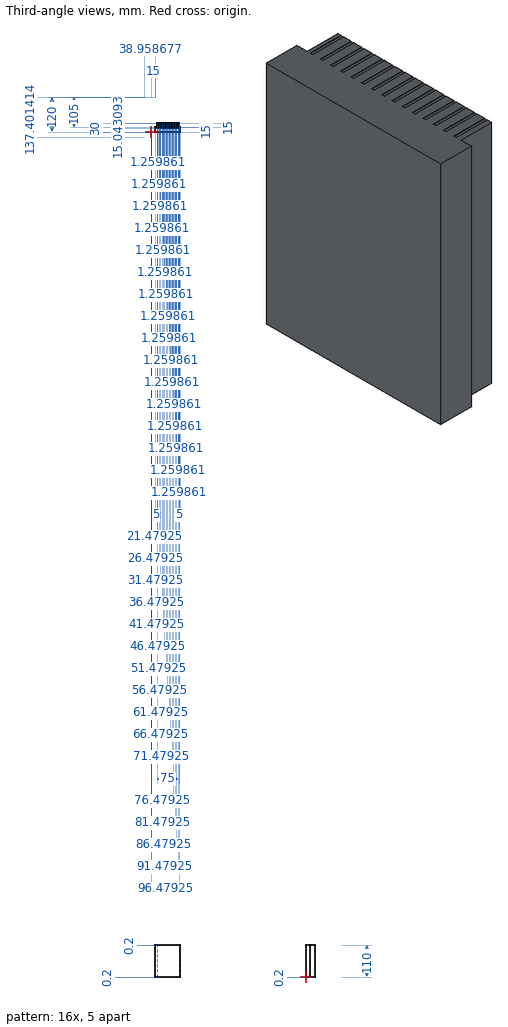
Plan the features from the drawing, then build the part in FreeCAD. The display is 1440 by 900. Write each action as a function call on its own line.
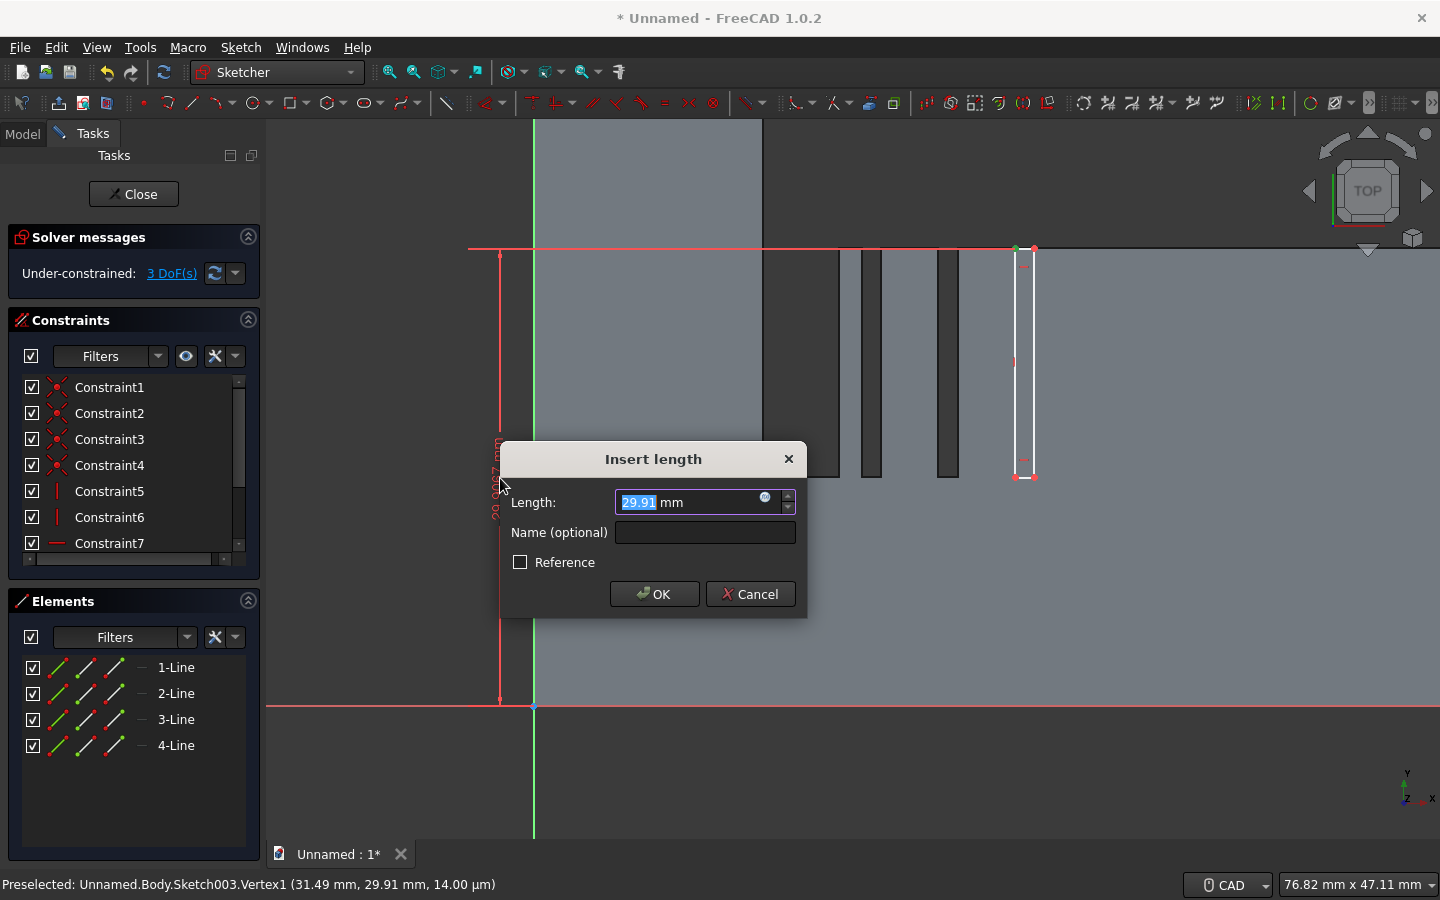
text(30)
key(Return)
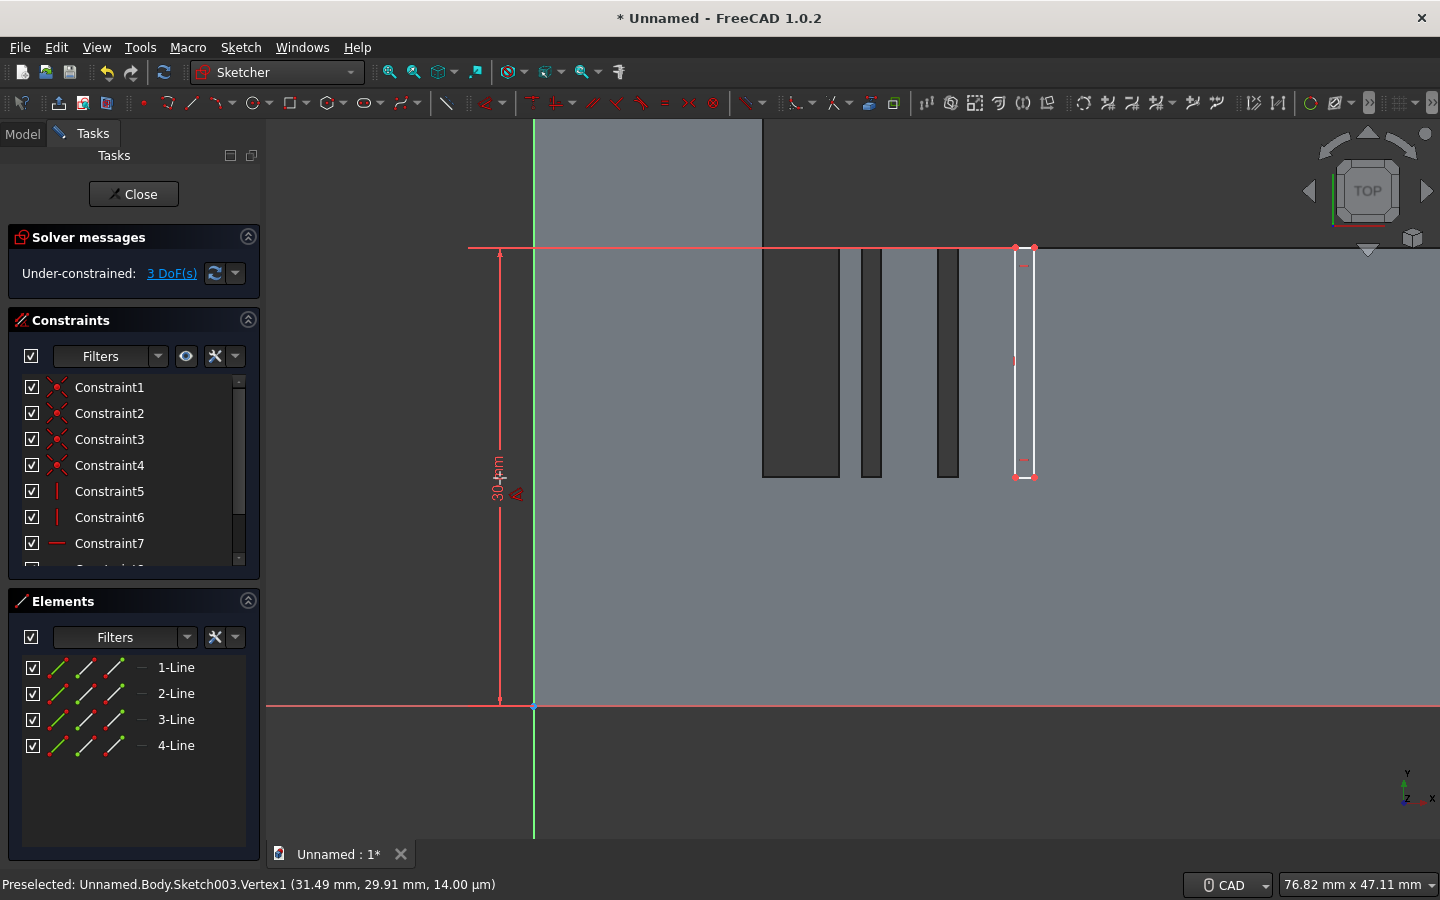
scroll(1025, 478, up, 4)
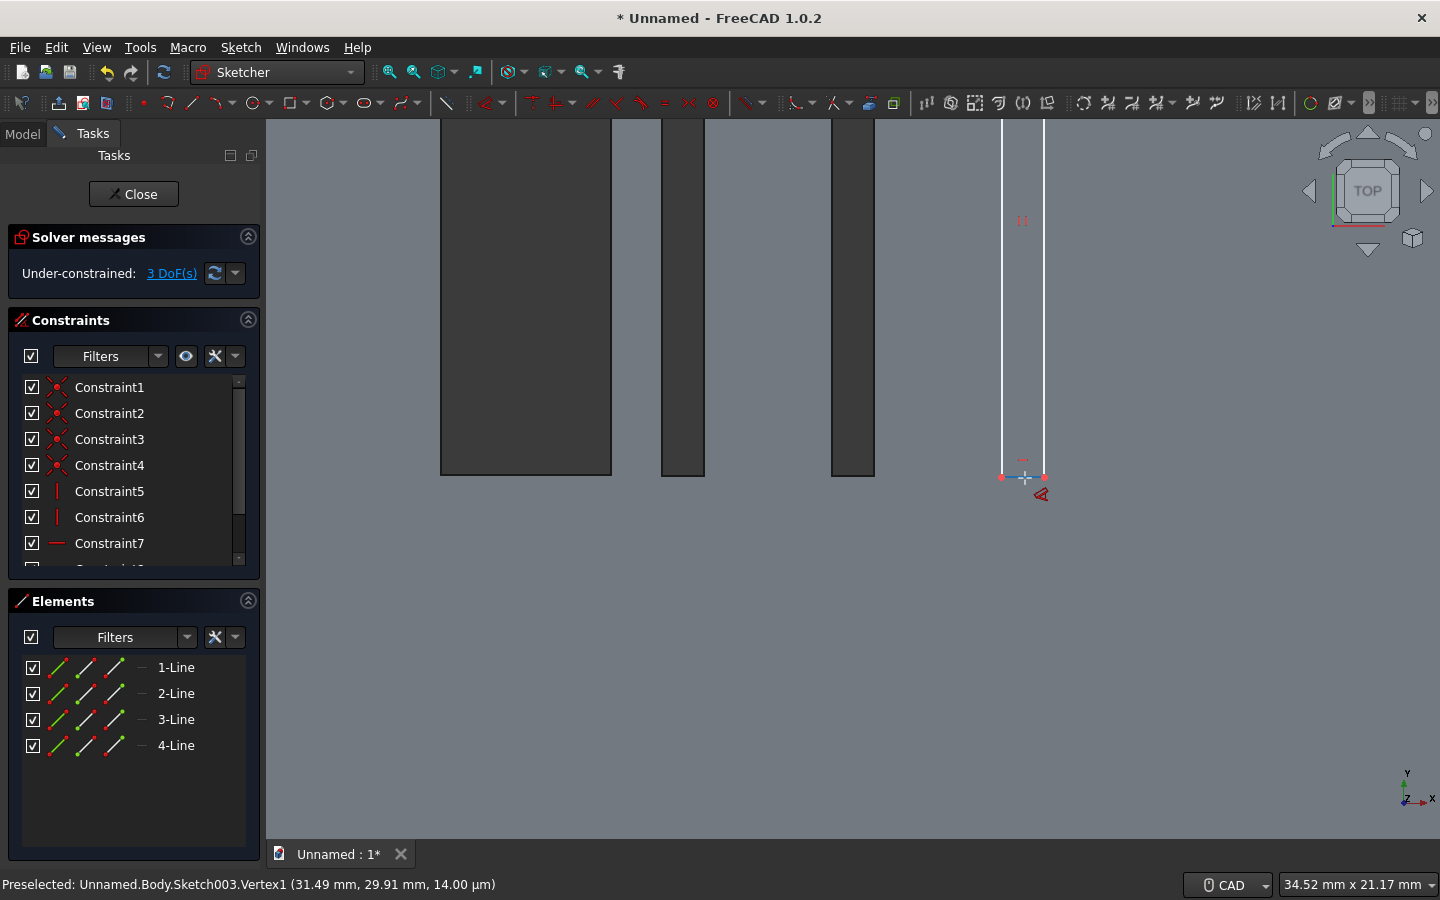
click(1023, 477)
click(1023, 511)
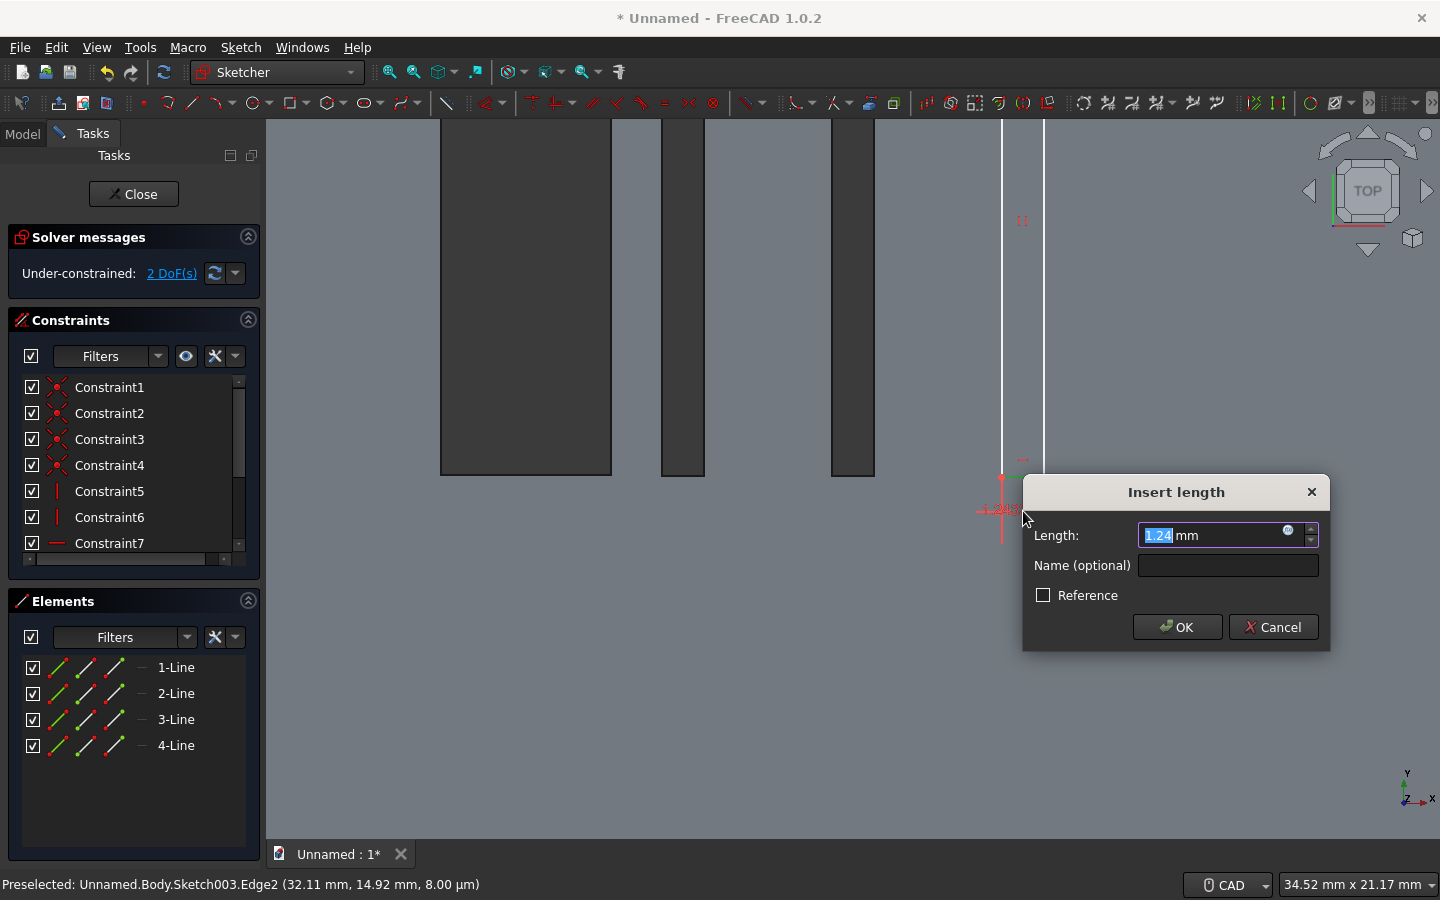
text(1.259861)
key(Return)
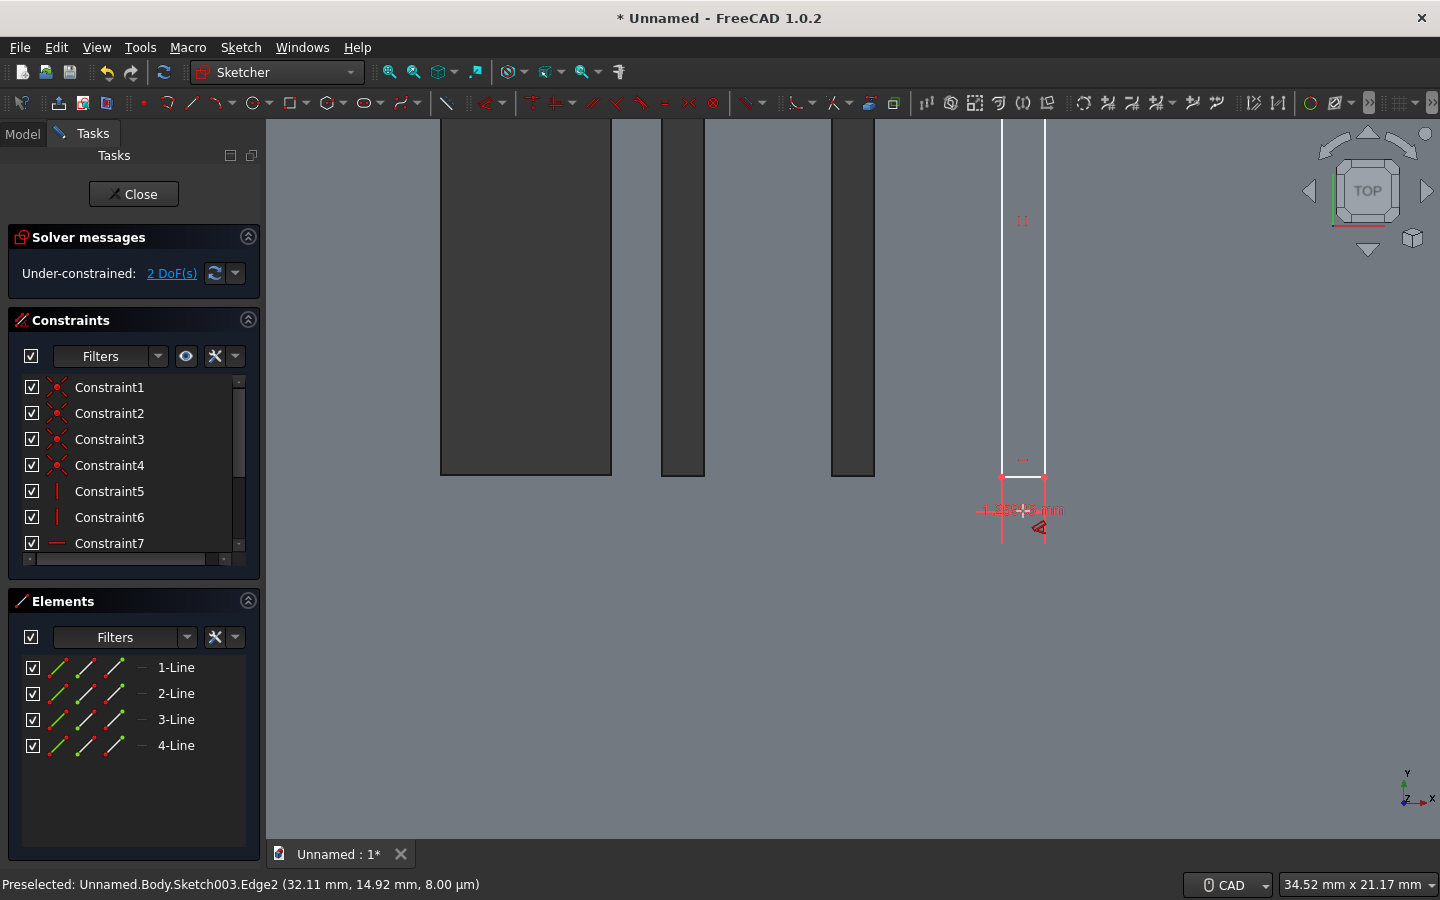
click(1002, 324)
click(968, 312)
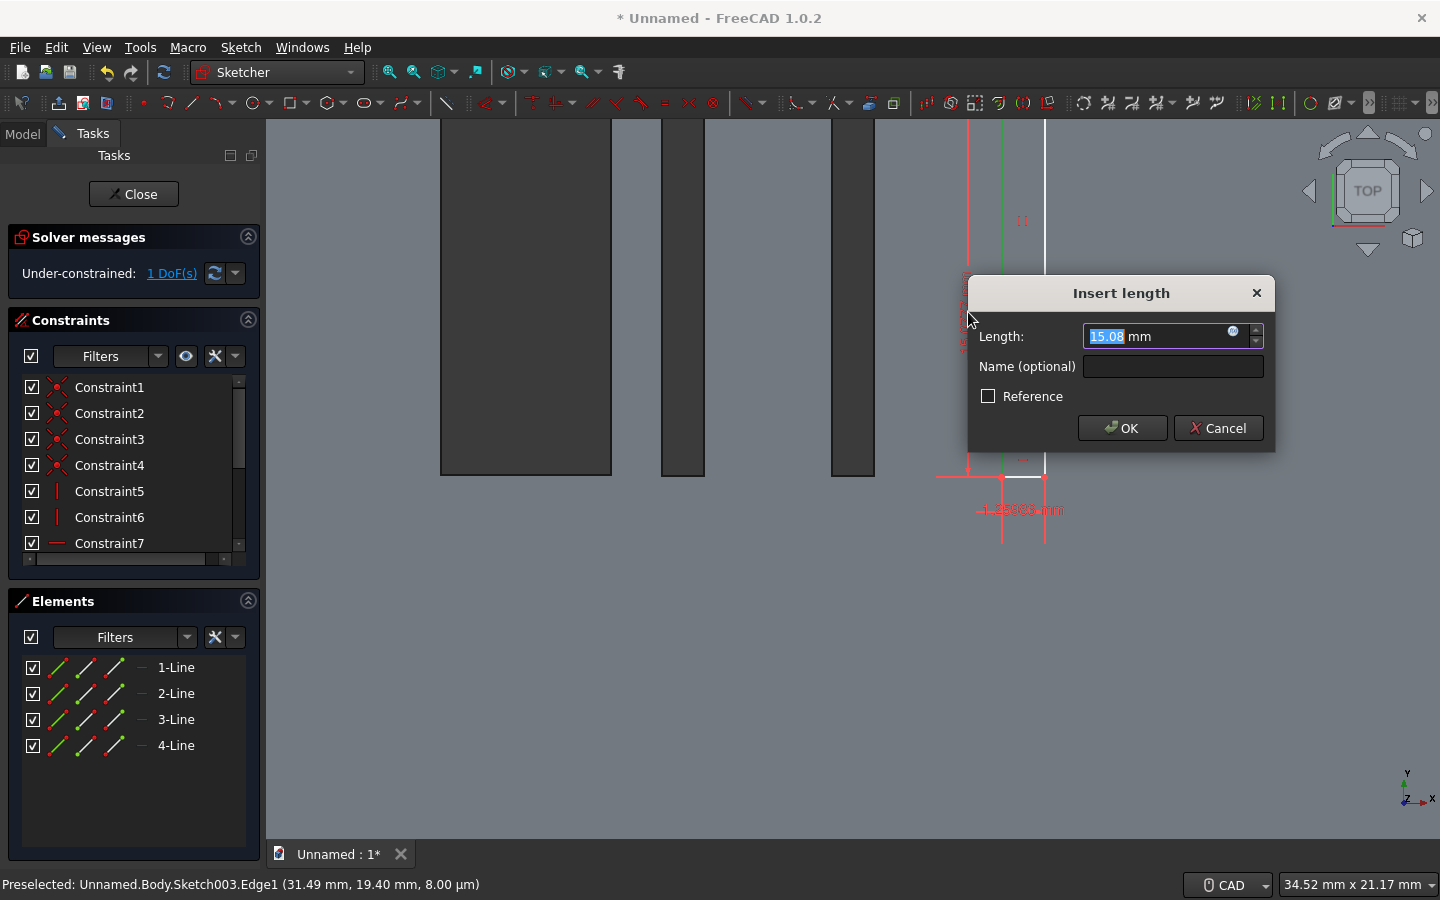
text(15.043093)
key(Return)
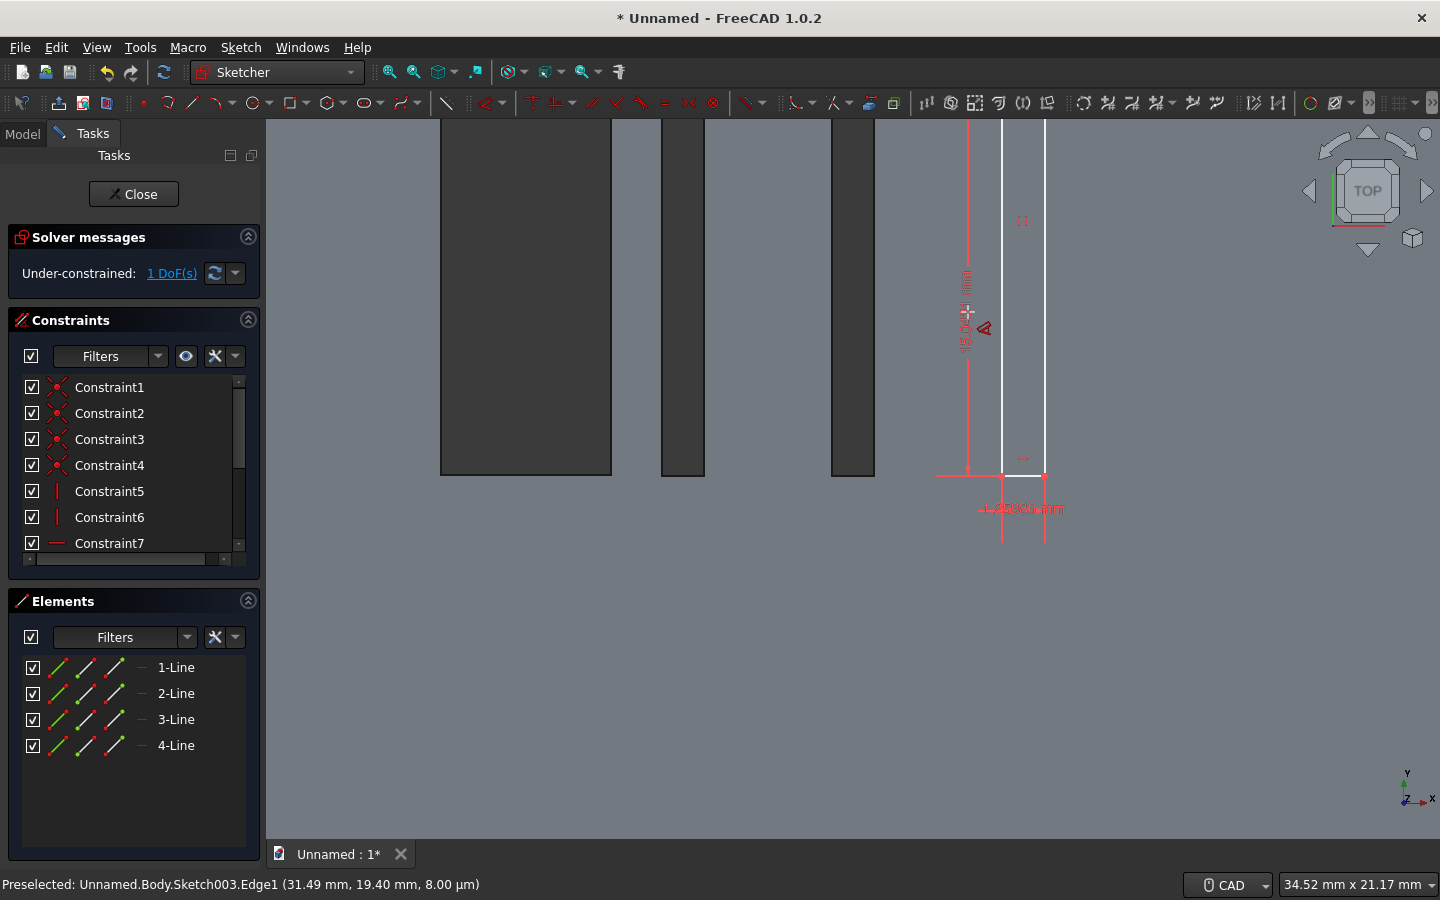
scroll(1027, 482, down, 4)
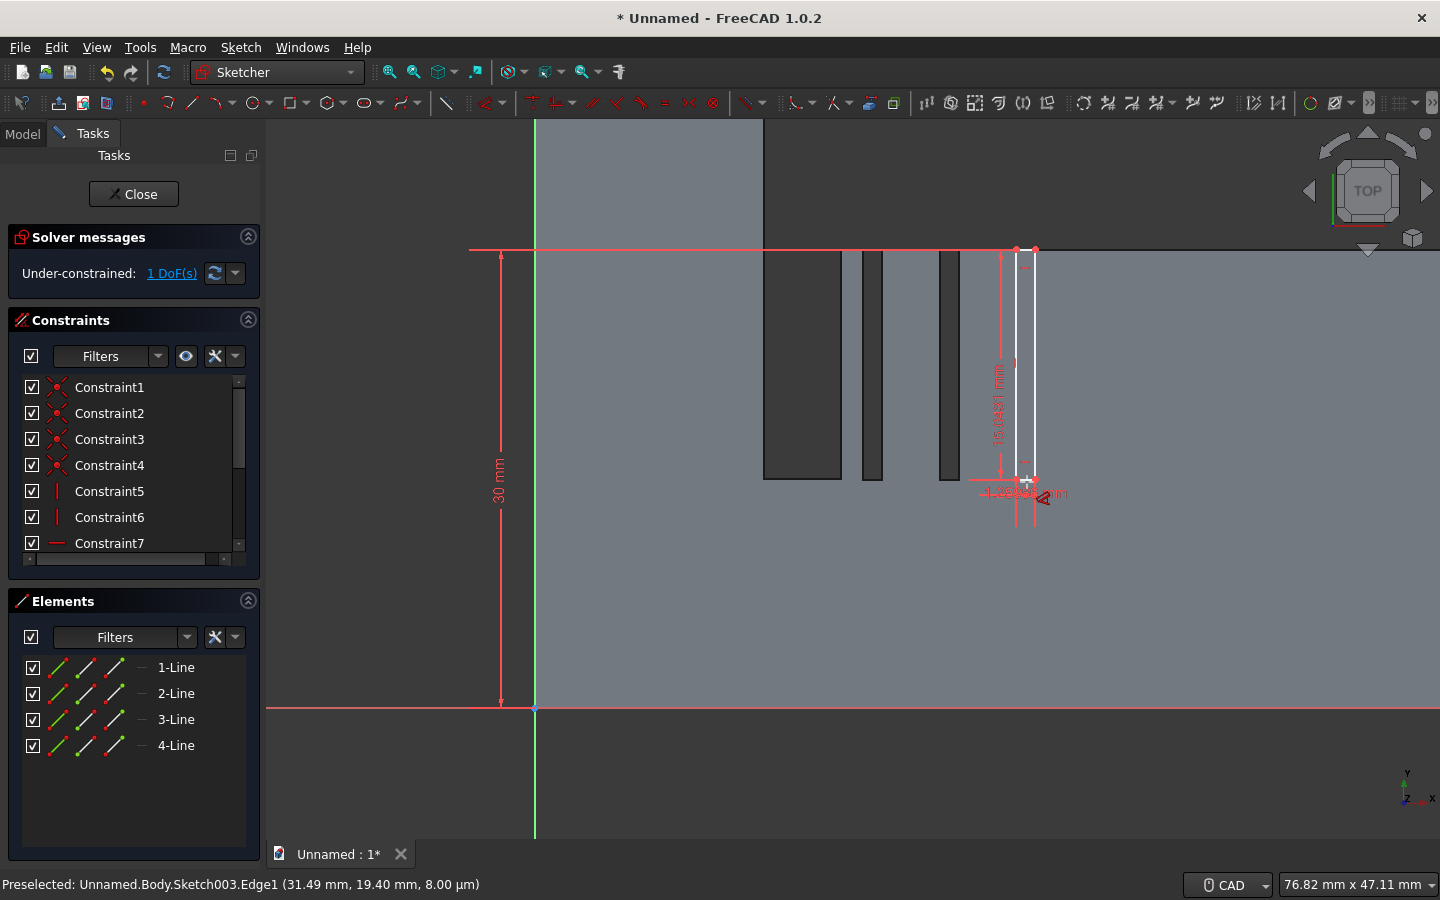
click(1016, 250)
click(775, 742)